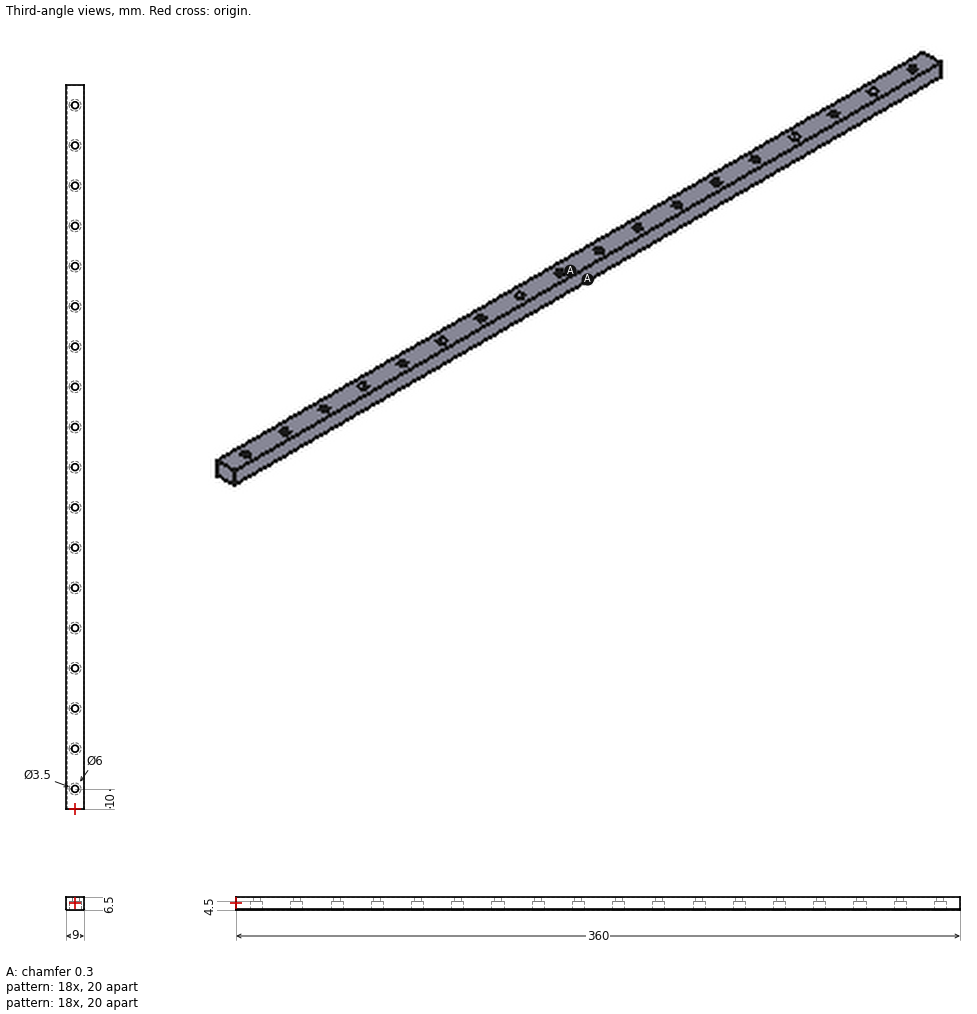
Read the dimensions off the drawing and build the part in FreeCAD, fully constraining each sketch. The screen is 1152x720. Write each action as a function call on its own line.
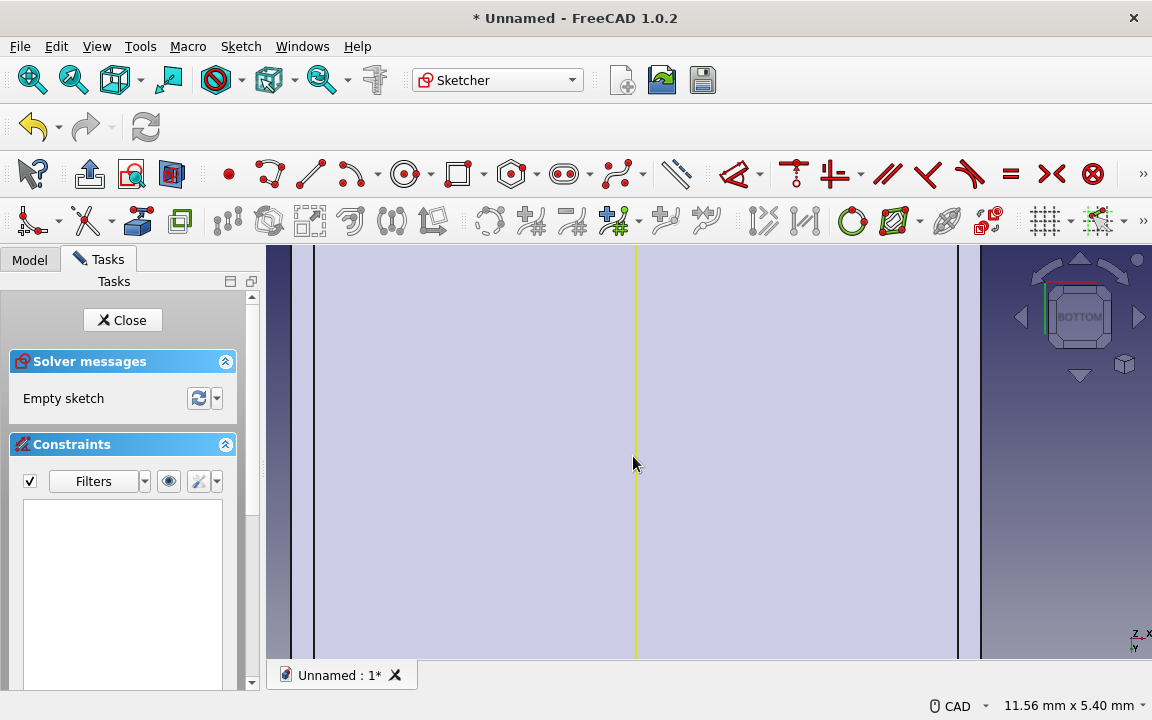
click(404, 174)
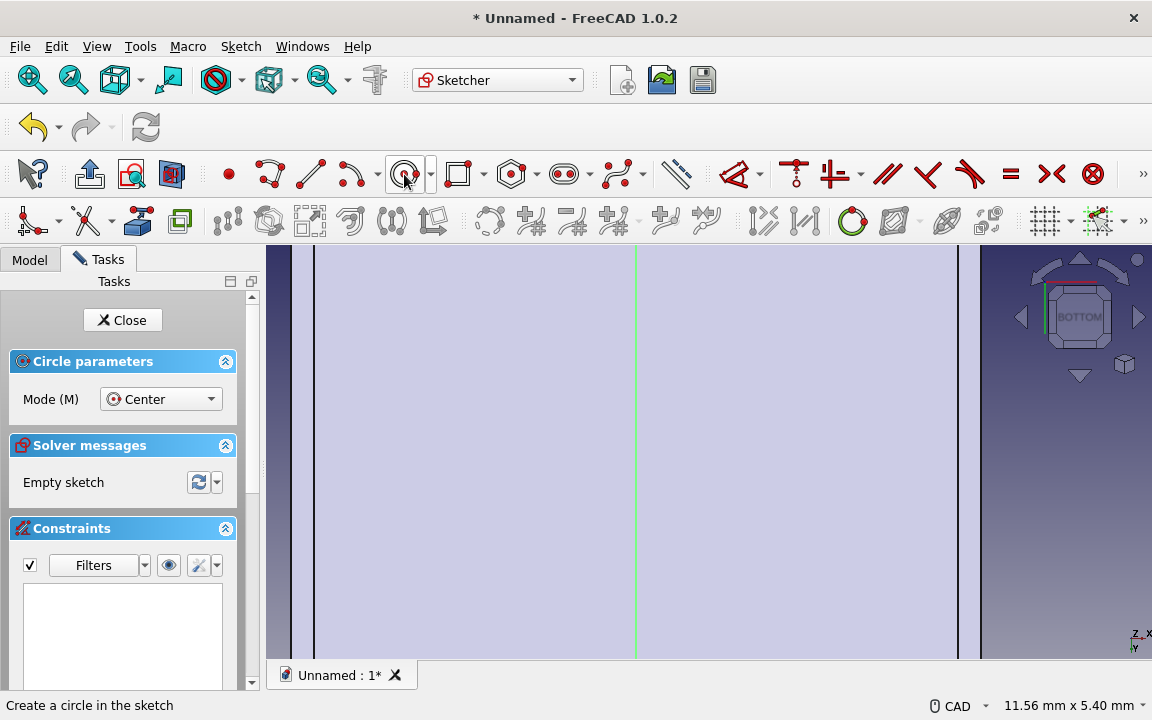
click(636, 450)
move(731, 355)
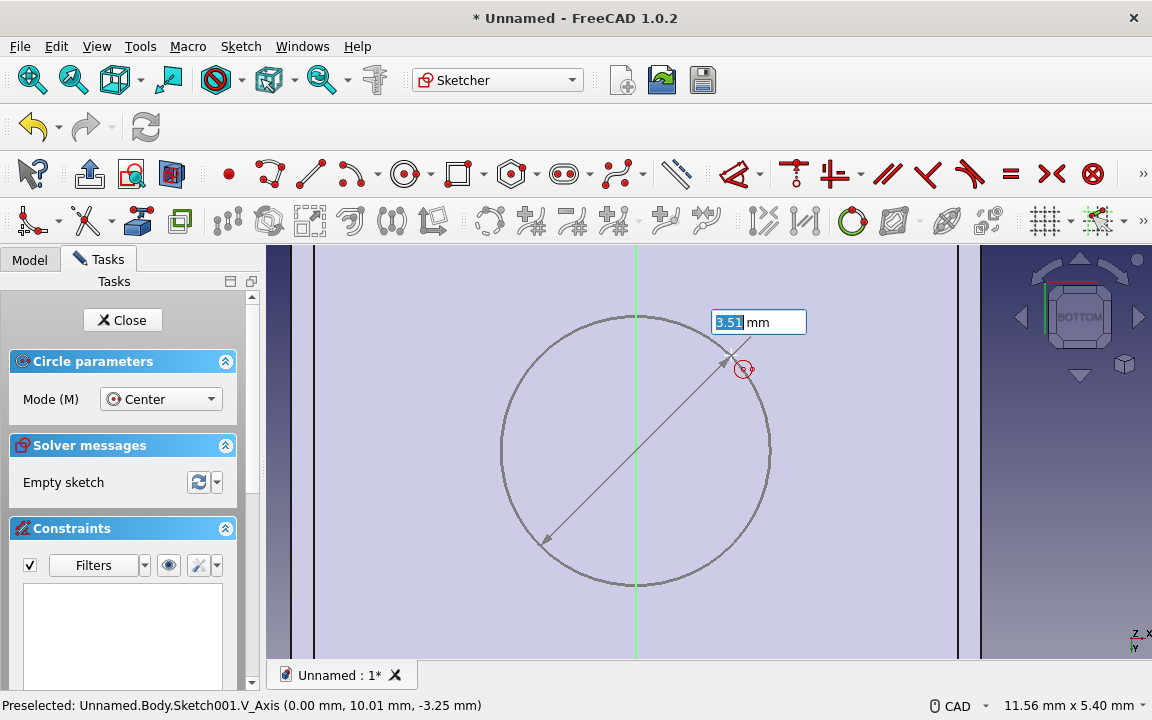
text(3.5)
key(Return)
key(Escape)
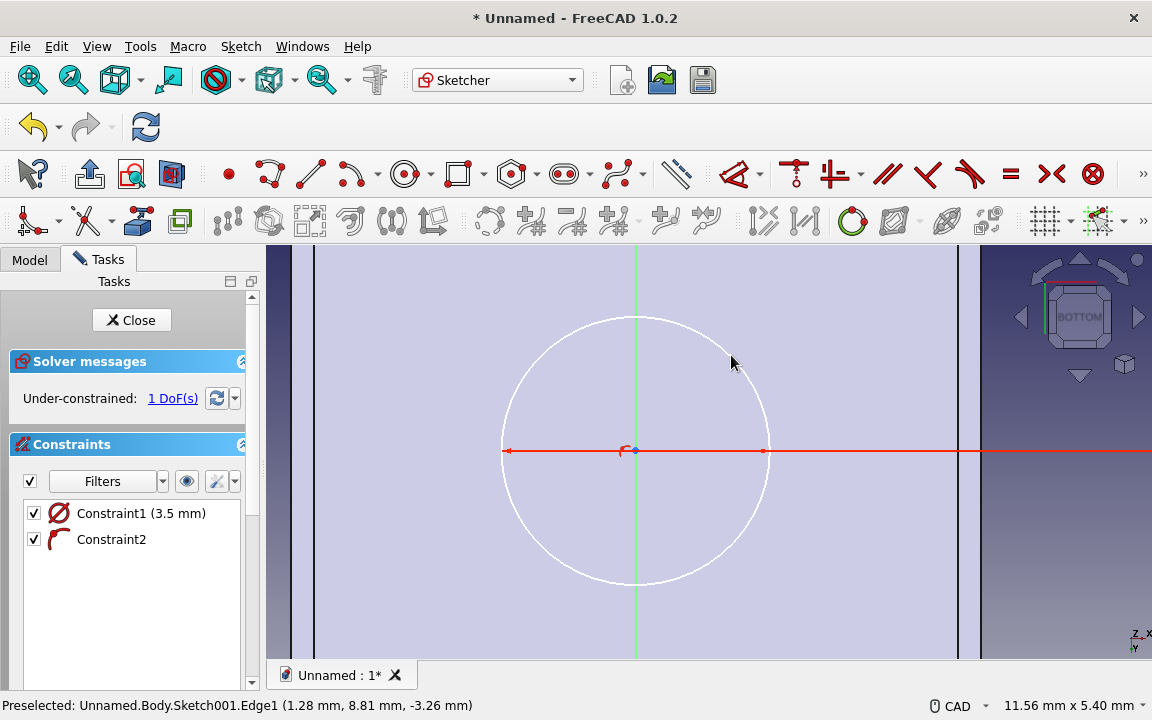
click(734, 174)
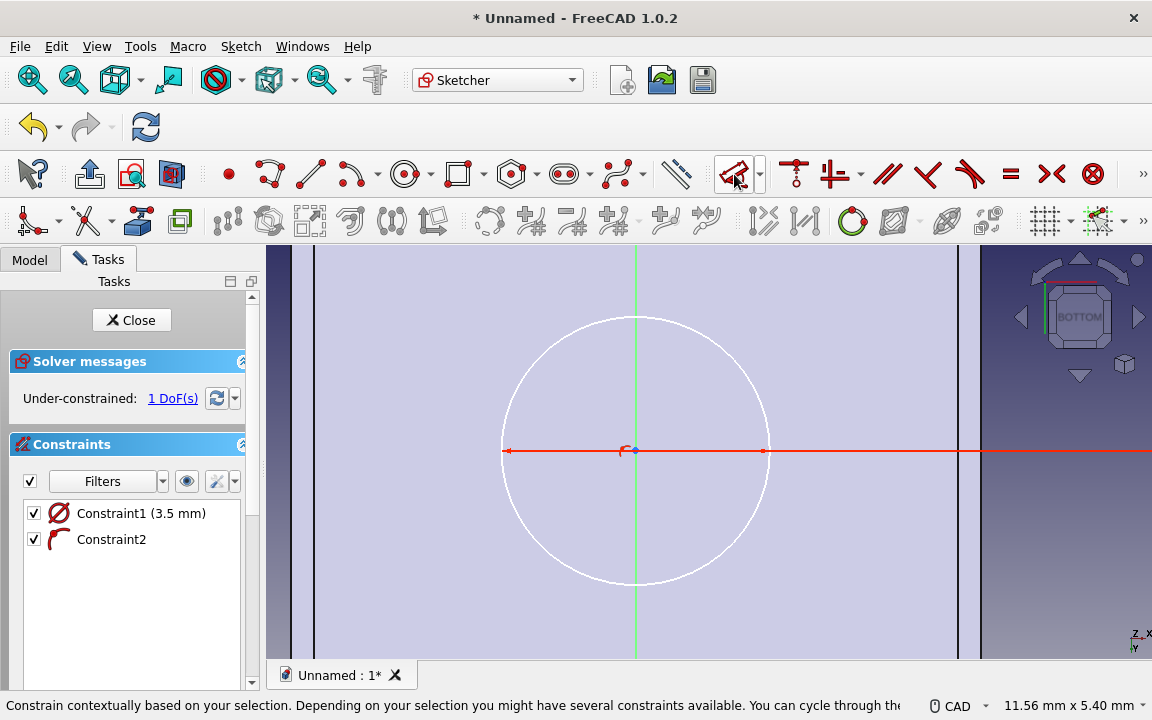
click(636, 451)
click(670, 362)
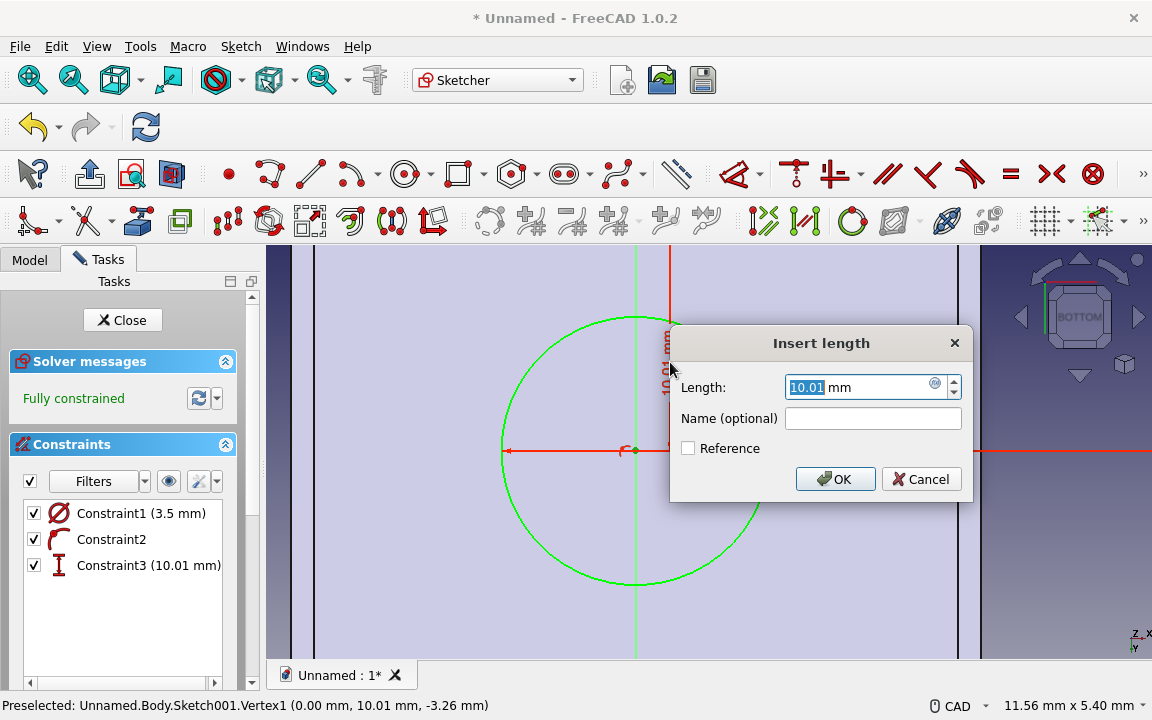
text(10)
key(Return)
key(Escape)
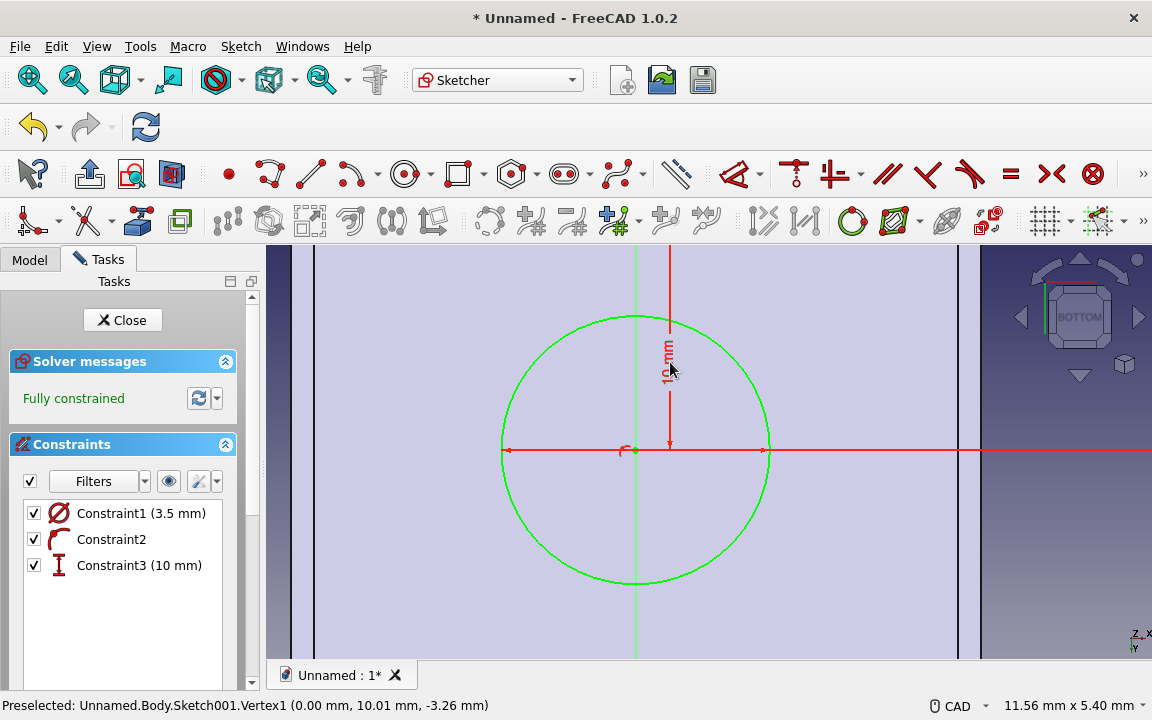
click(123, 320)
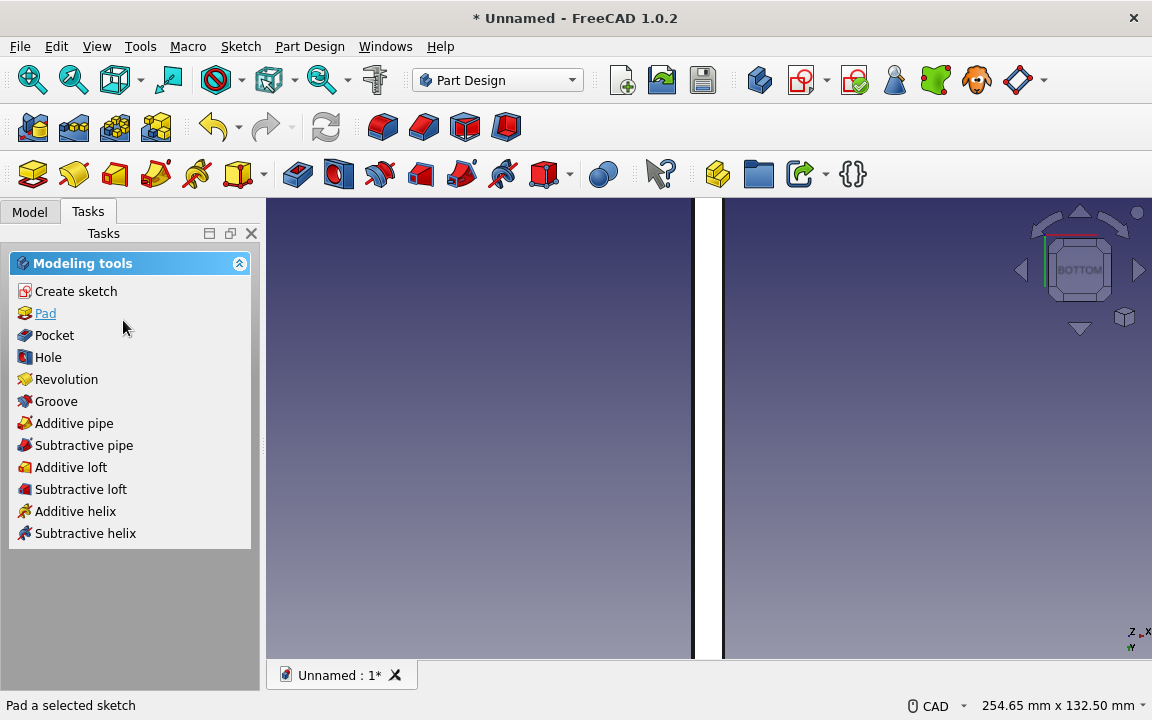
click(298, 174)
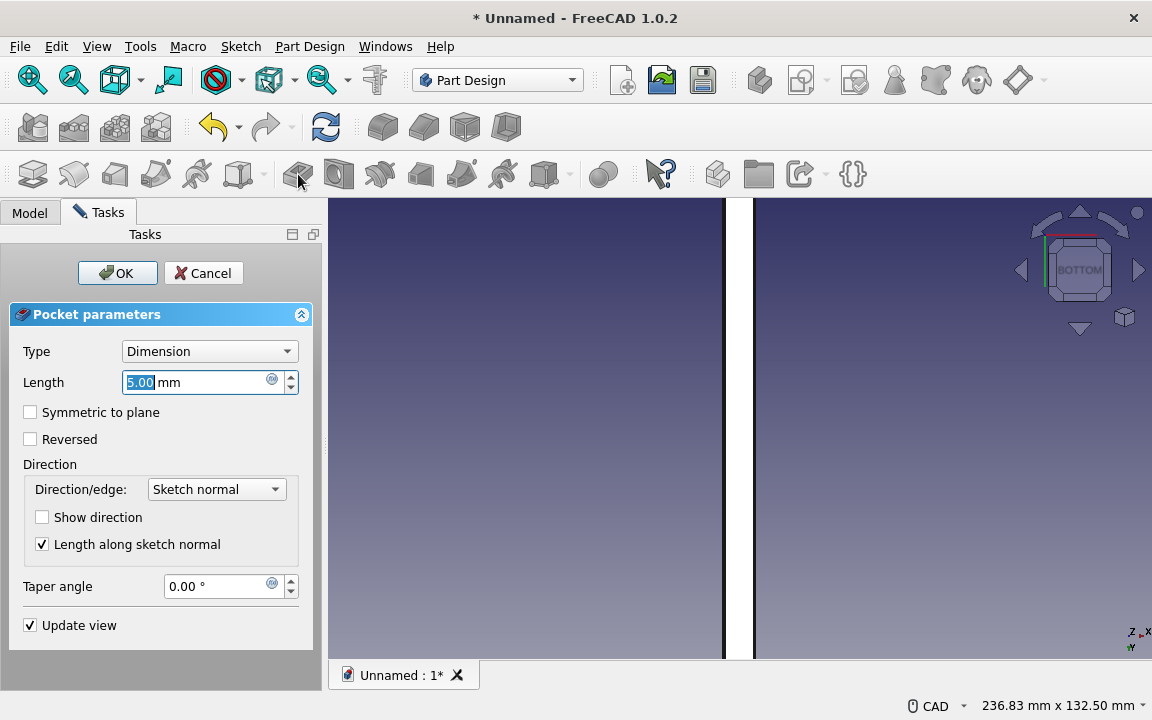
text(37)
key(Tab)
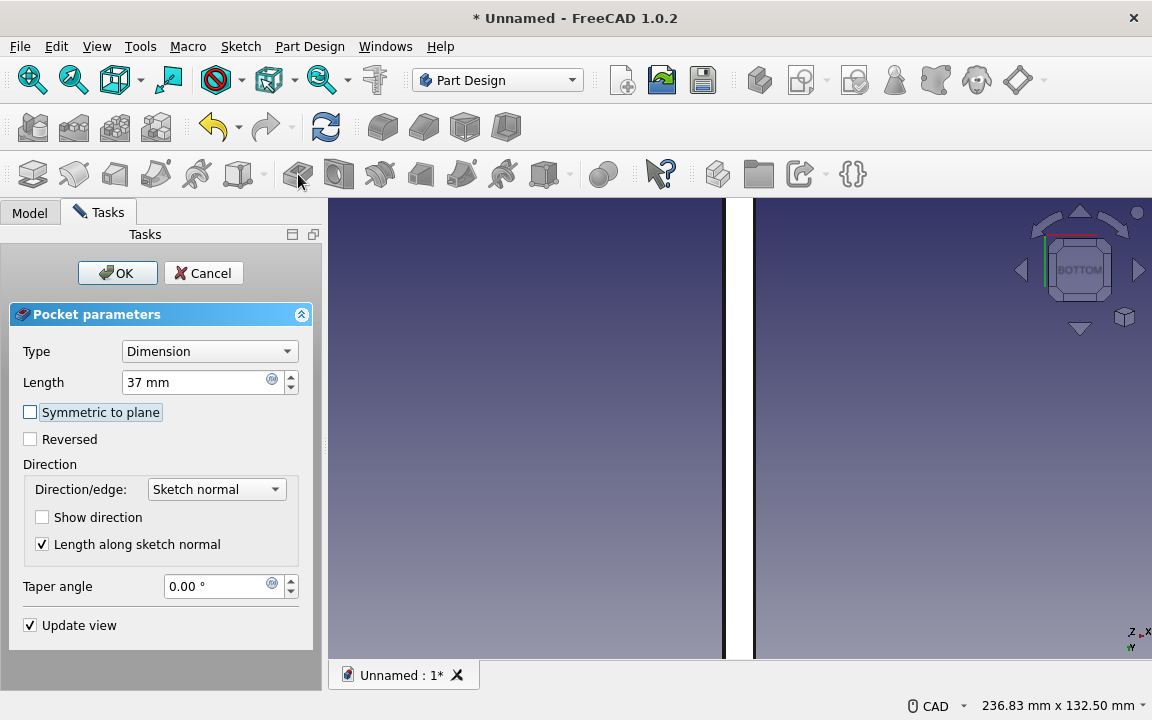
click(118, 273)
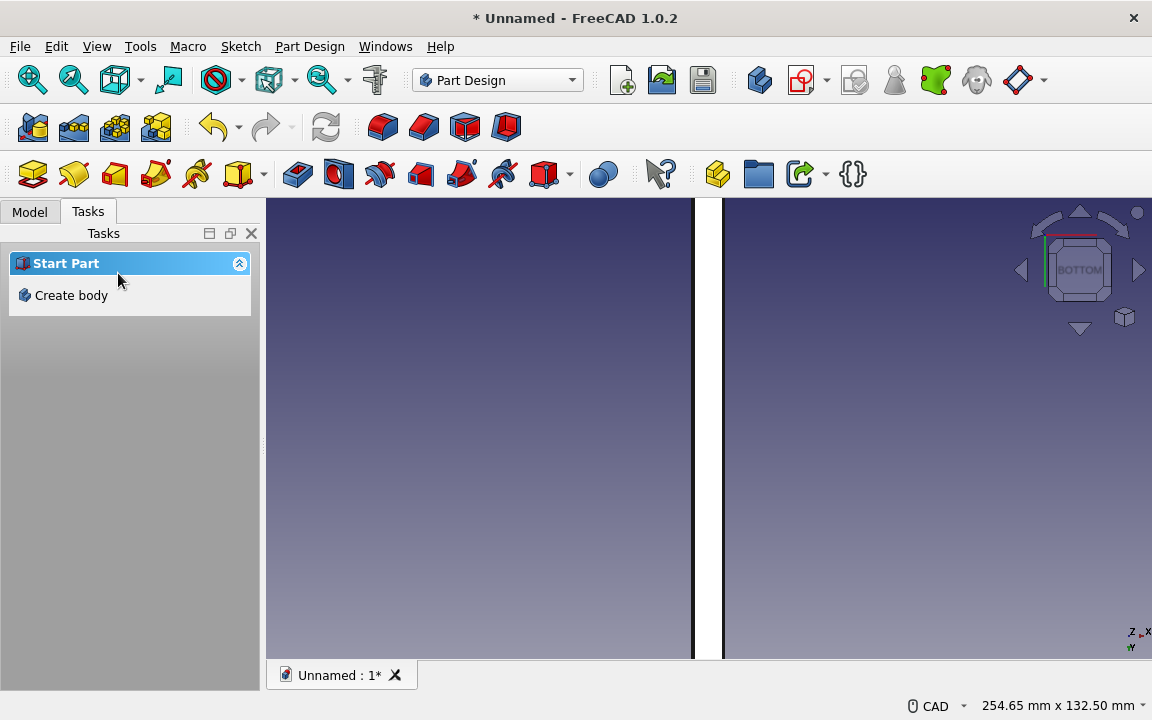
key(v)
key(f)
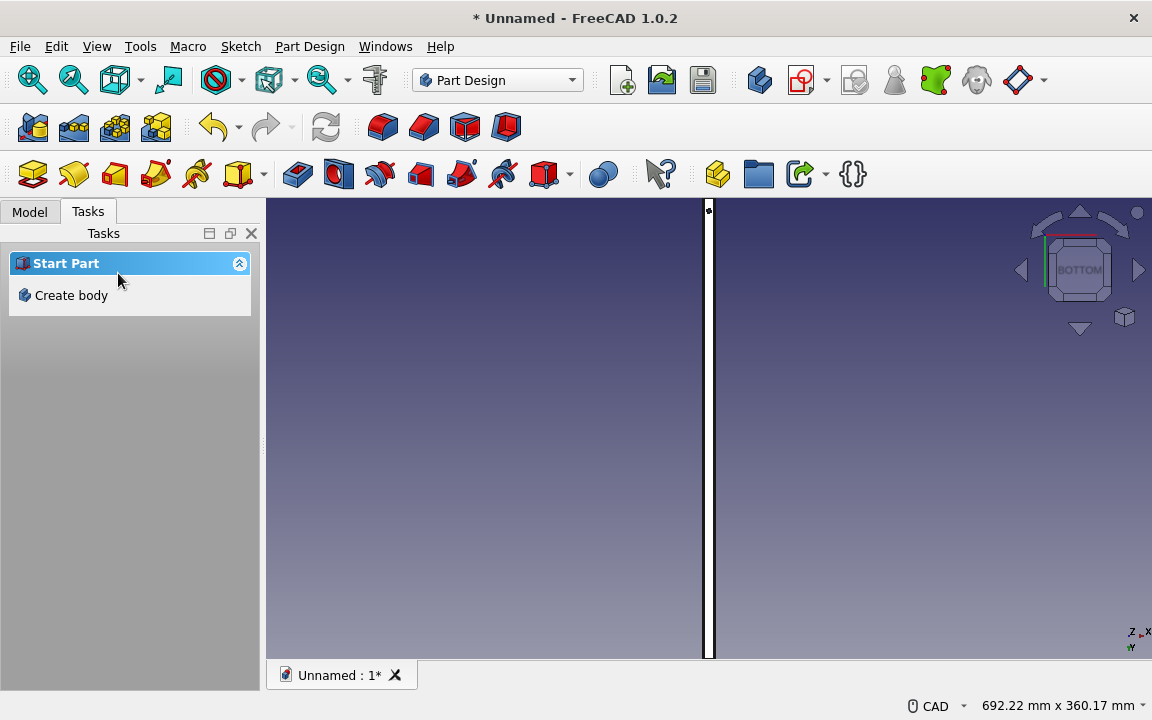
click(30, 212)